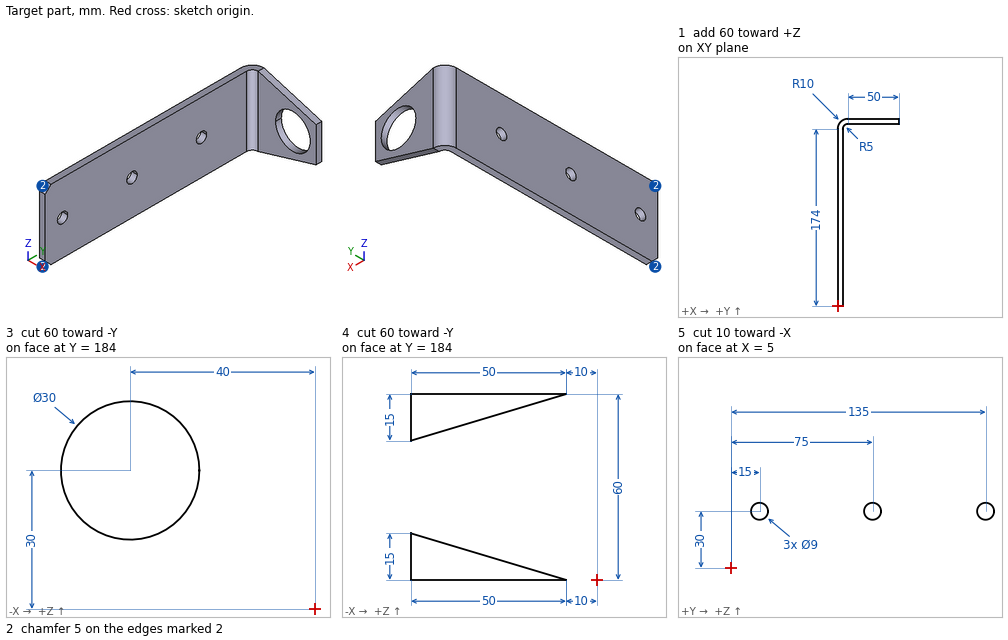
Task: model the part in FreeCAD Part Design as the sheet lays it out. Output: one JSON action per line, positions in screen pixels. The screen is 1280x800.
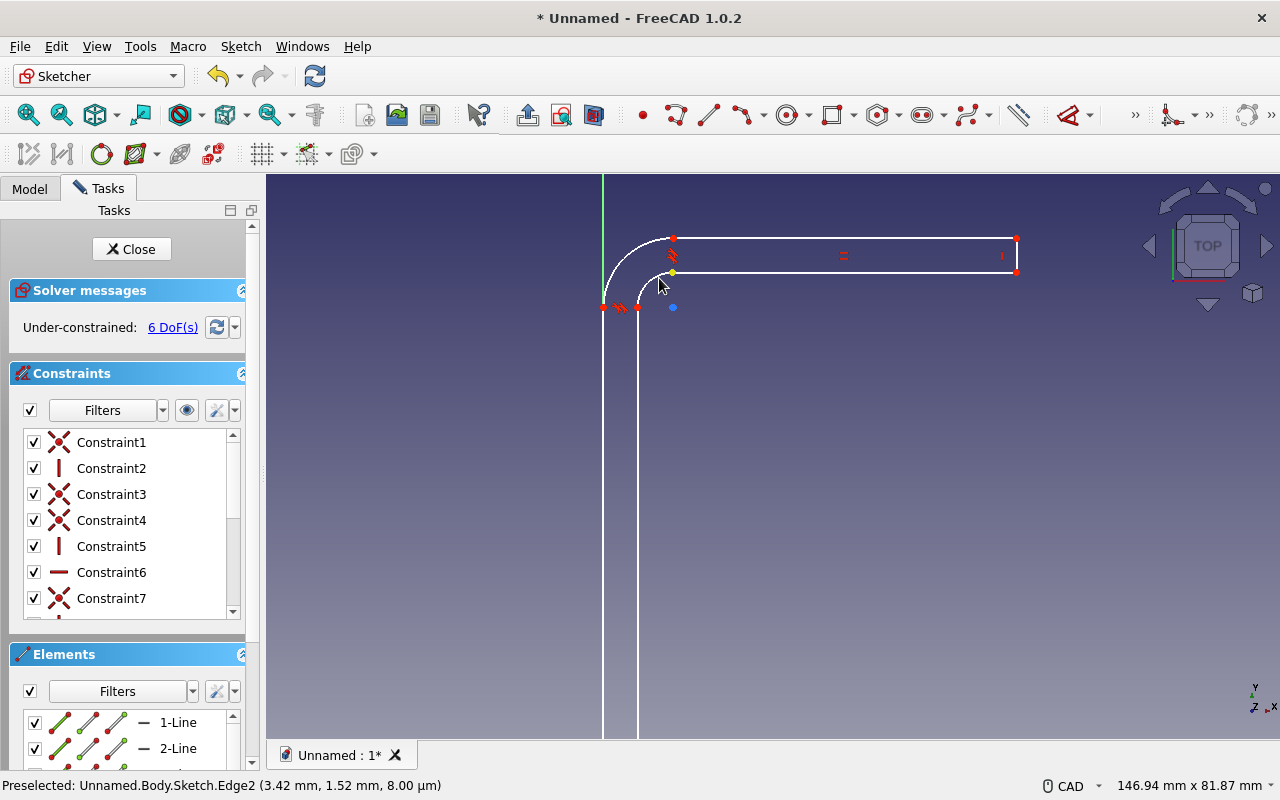
{"action": "left_click", "coordinate": [657, 277]}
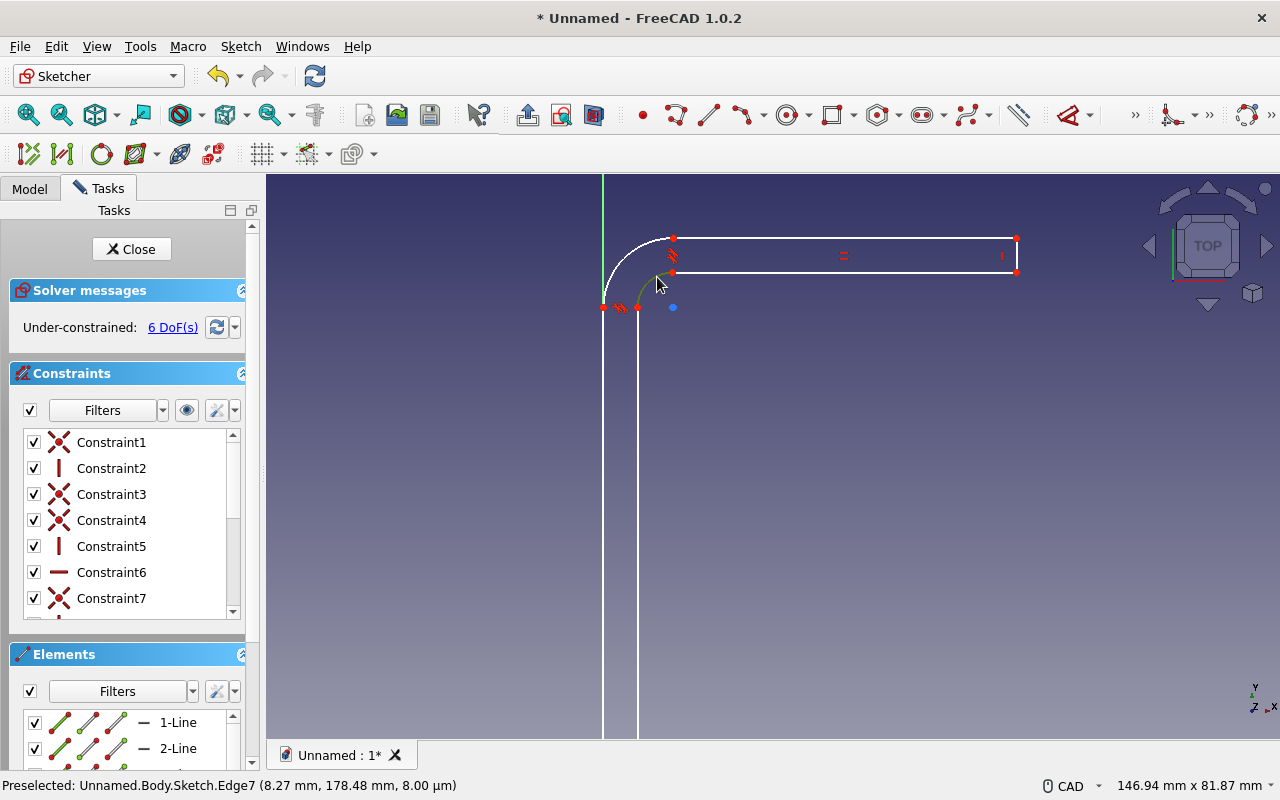
{"action": "left_click", "coordinate": [642, 246]}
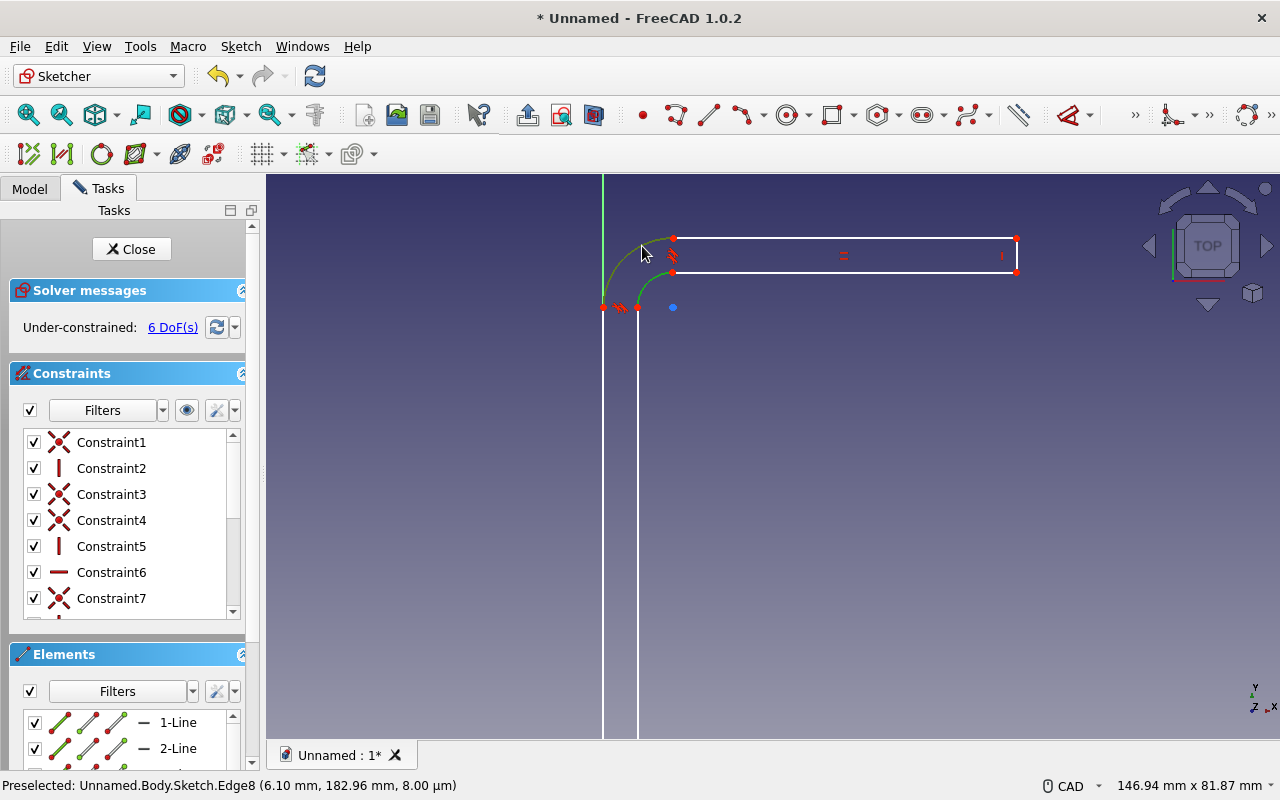
{"action": "key", "text": "c"}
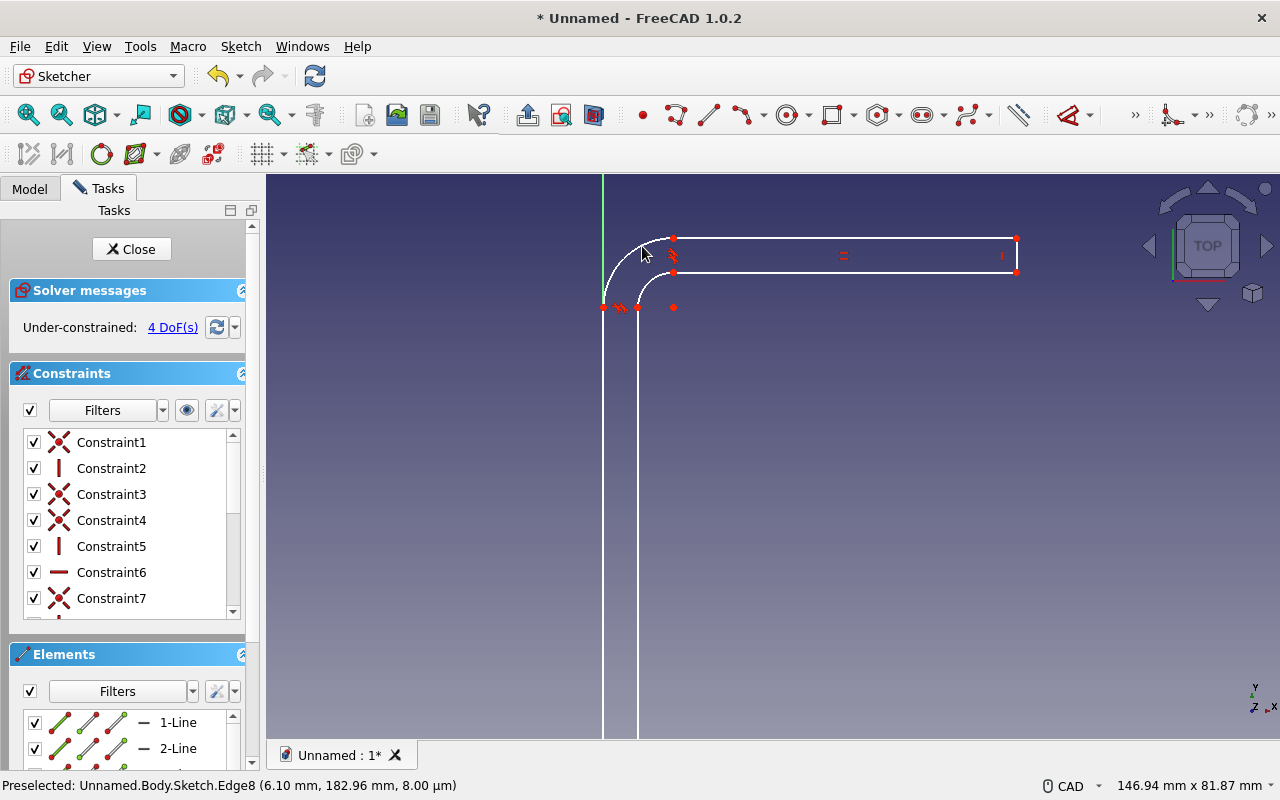
{"action": "key", "text": "d"}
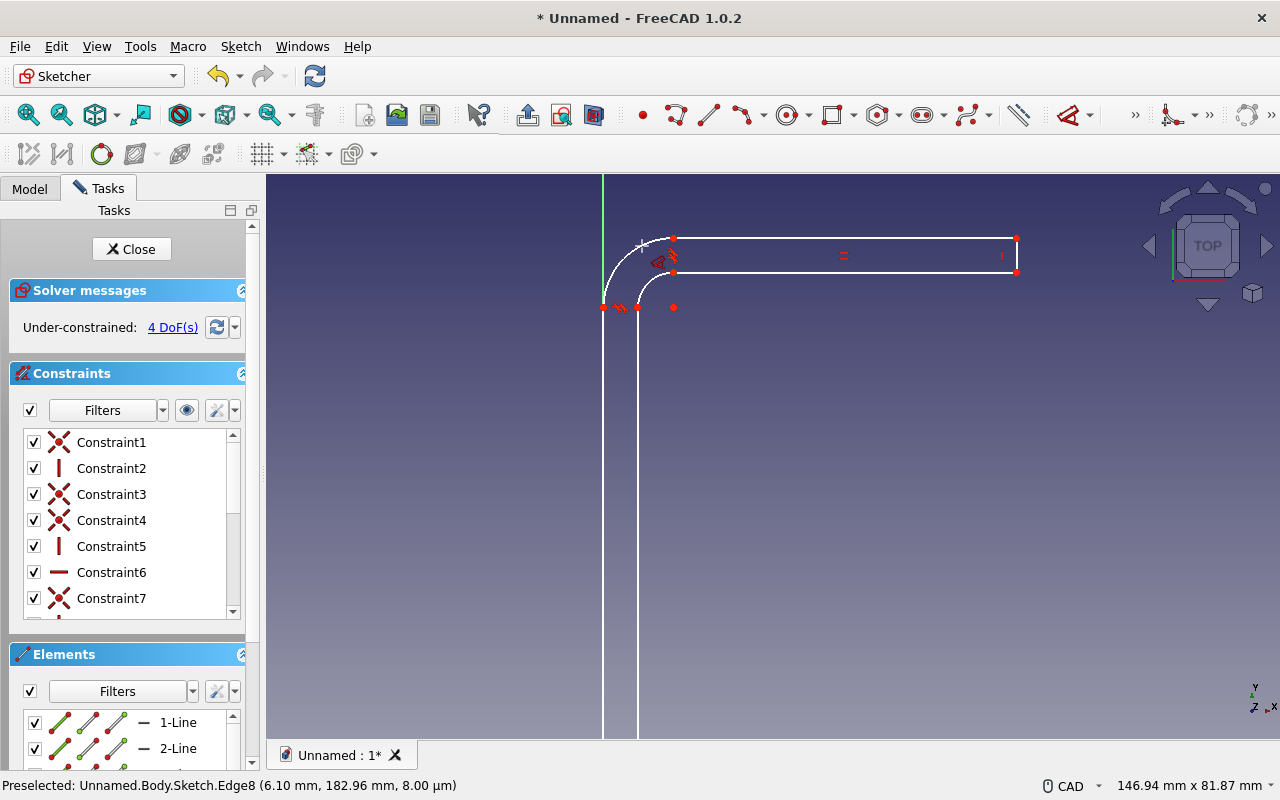
{"action": "left_click", "coordinate": [657, 276]}
{"action": "left_click", "coordinate": [704, 368]}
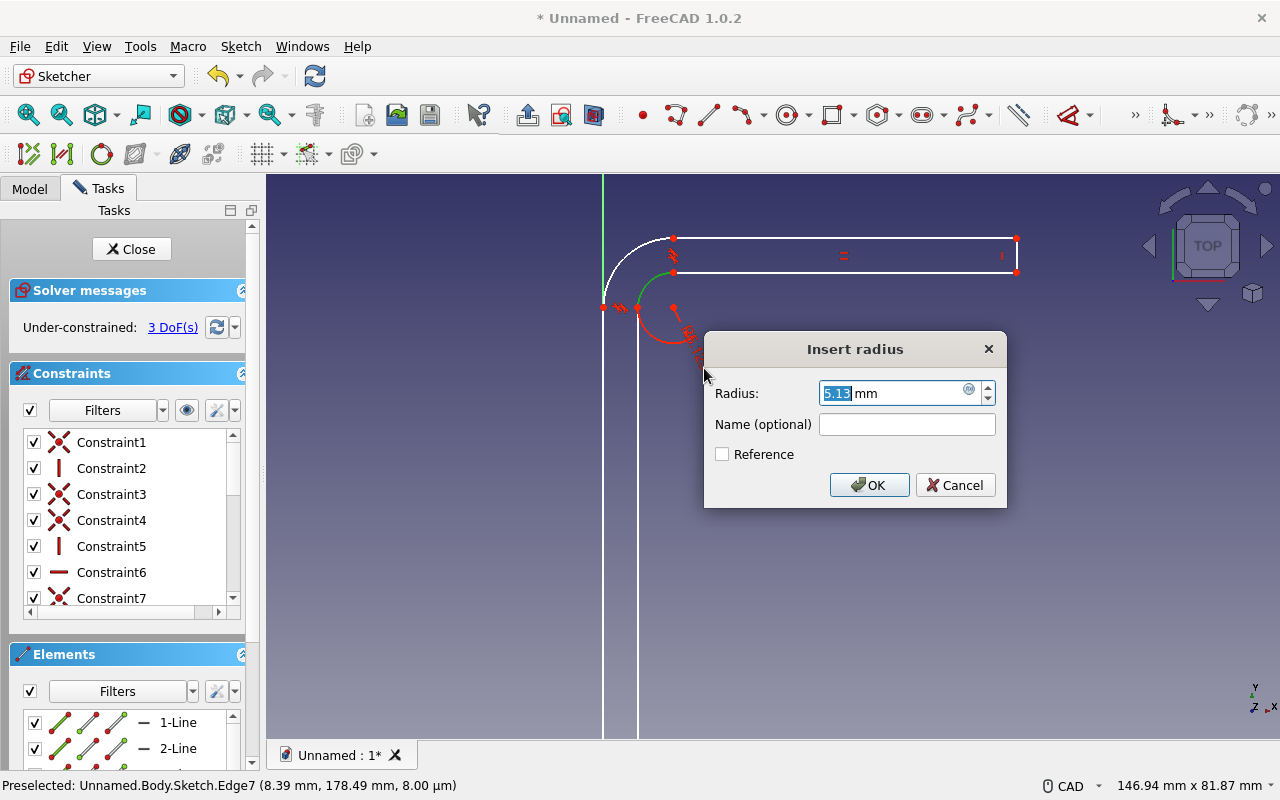
{"action": "type", "text": "5"}
{"action": "key", "text": "Return"}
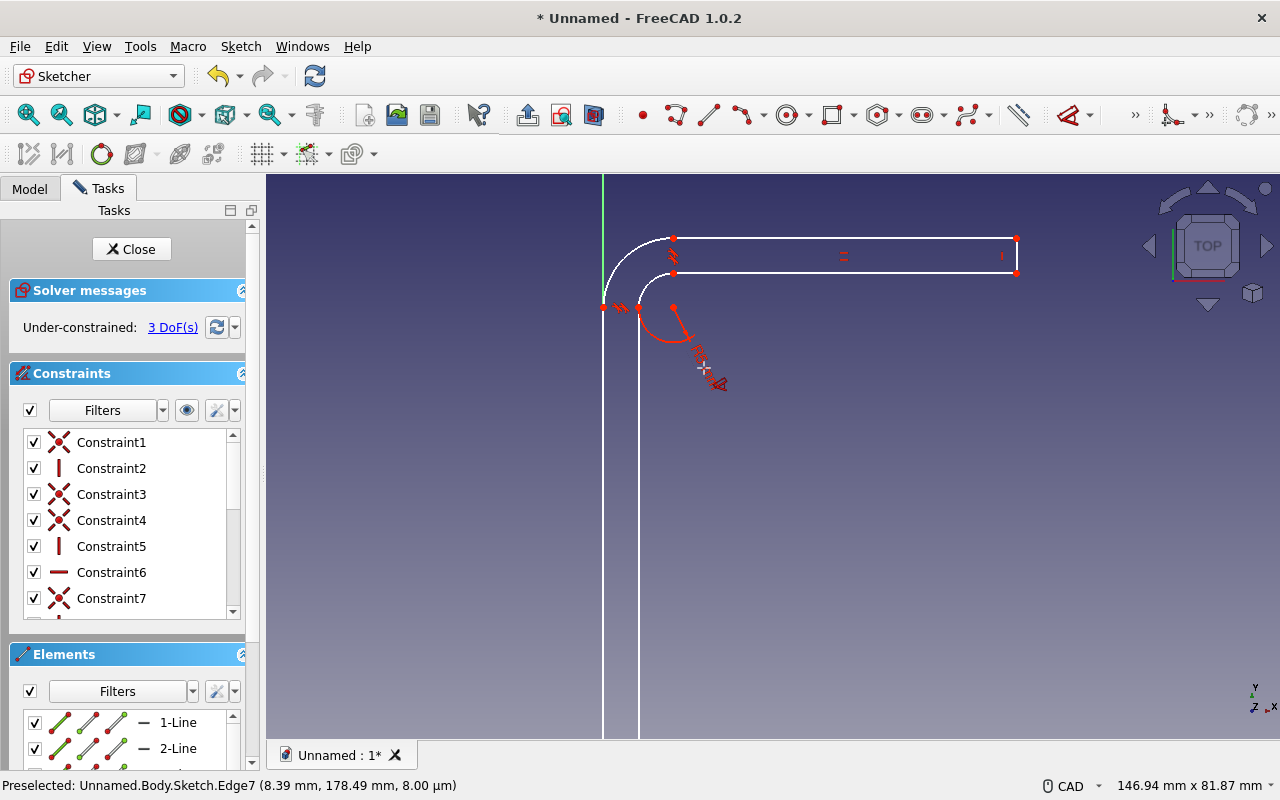
{"action": "left_click", "coordinate": [642, 246]}
{"action": "left_click", "coordinate": [628, 217]}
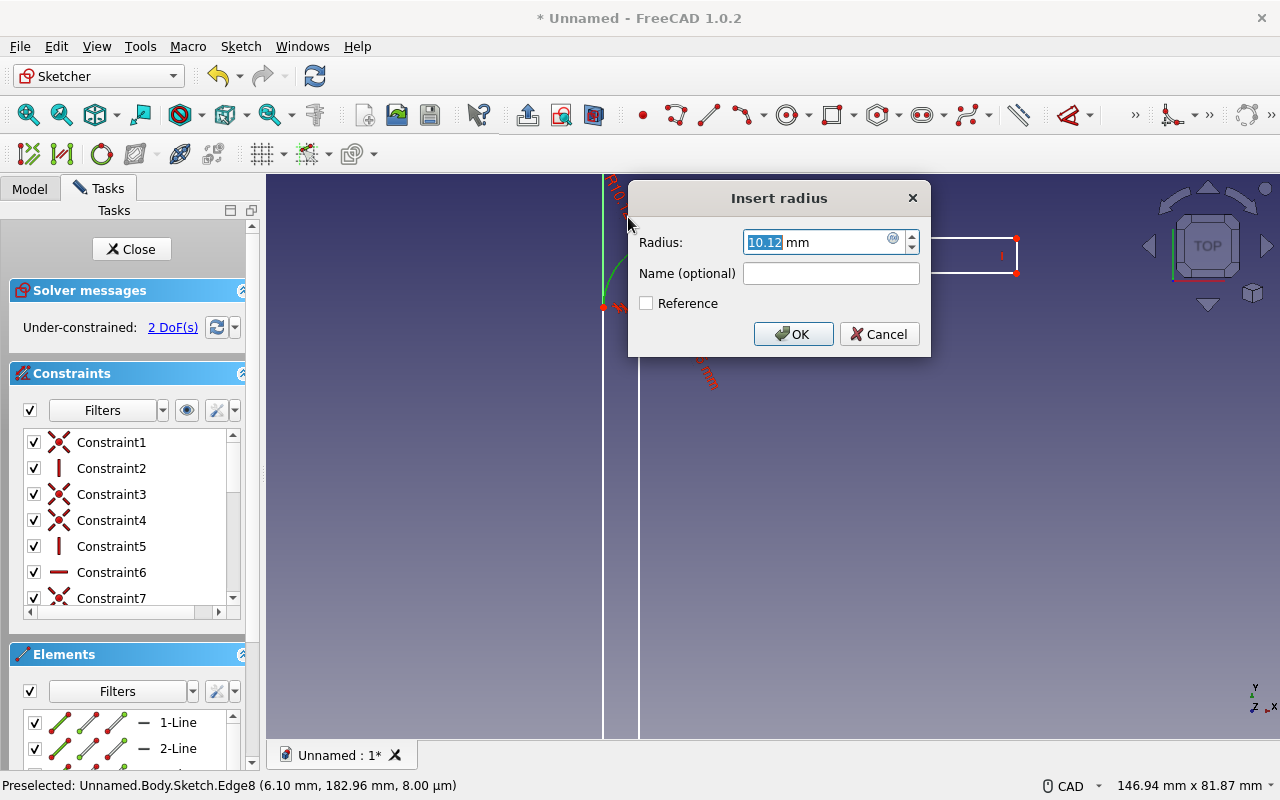
{"action": "type", "text": "10"}
{"action": "key", "text": "Return"}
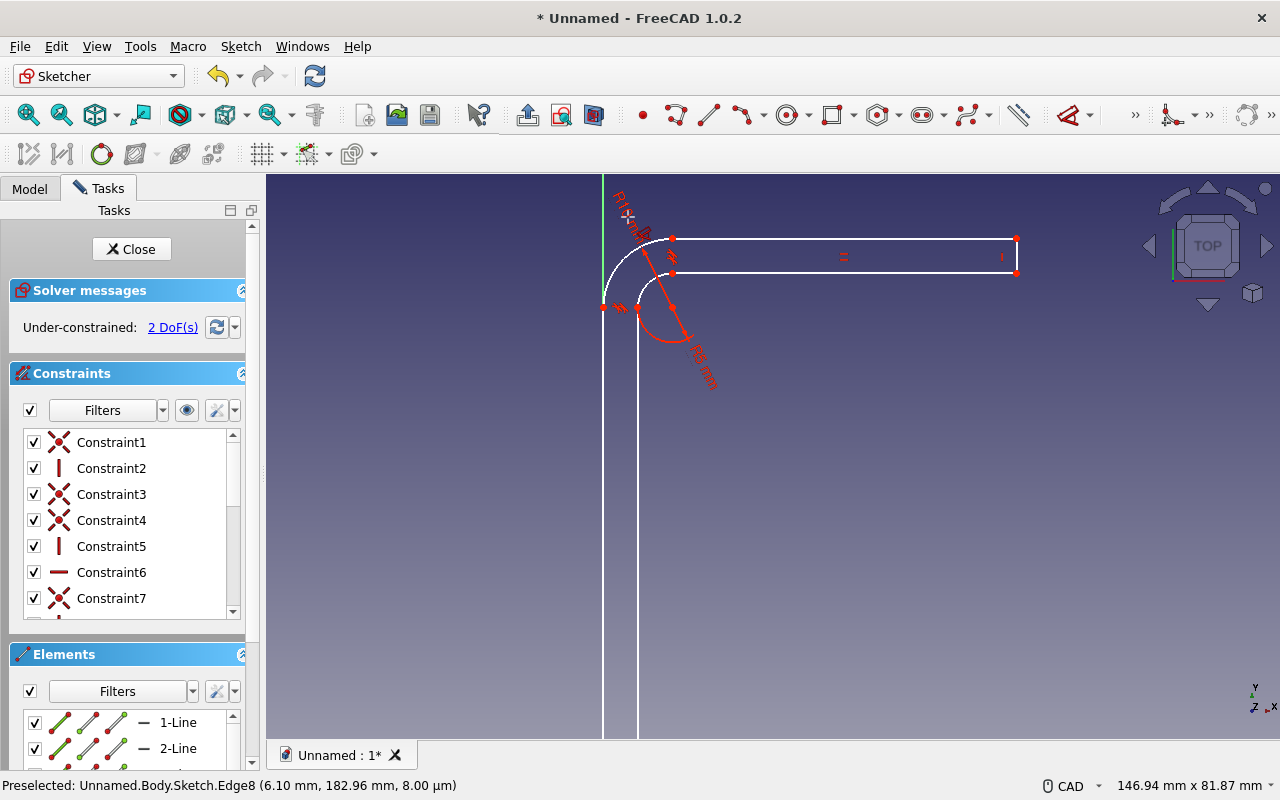
{"action": "left_click", "coordinate": [776, 273]}
{"action": "left_click", "coordinate": [845, 307]}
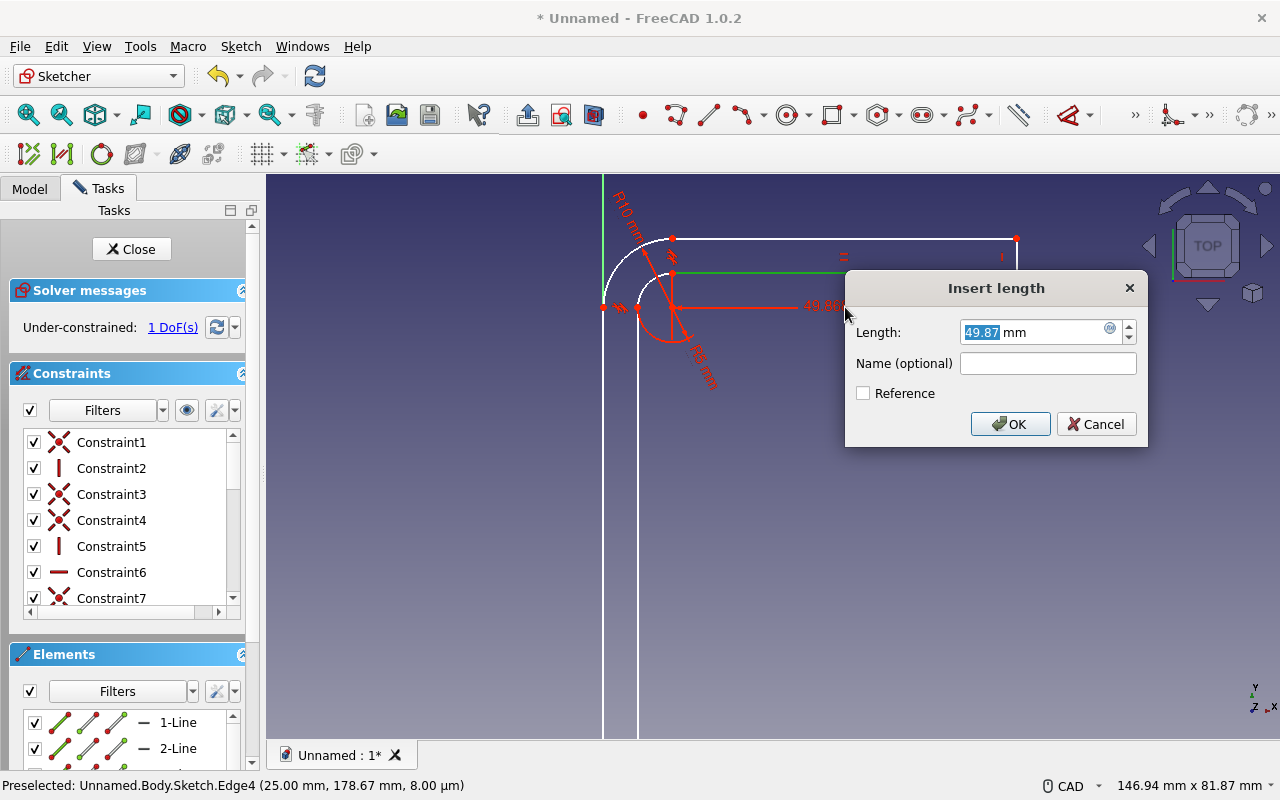
{"action": "type", "text": "50"}
{"action": "key", "text": "Return"}